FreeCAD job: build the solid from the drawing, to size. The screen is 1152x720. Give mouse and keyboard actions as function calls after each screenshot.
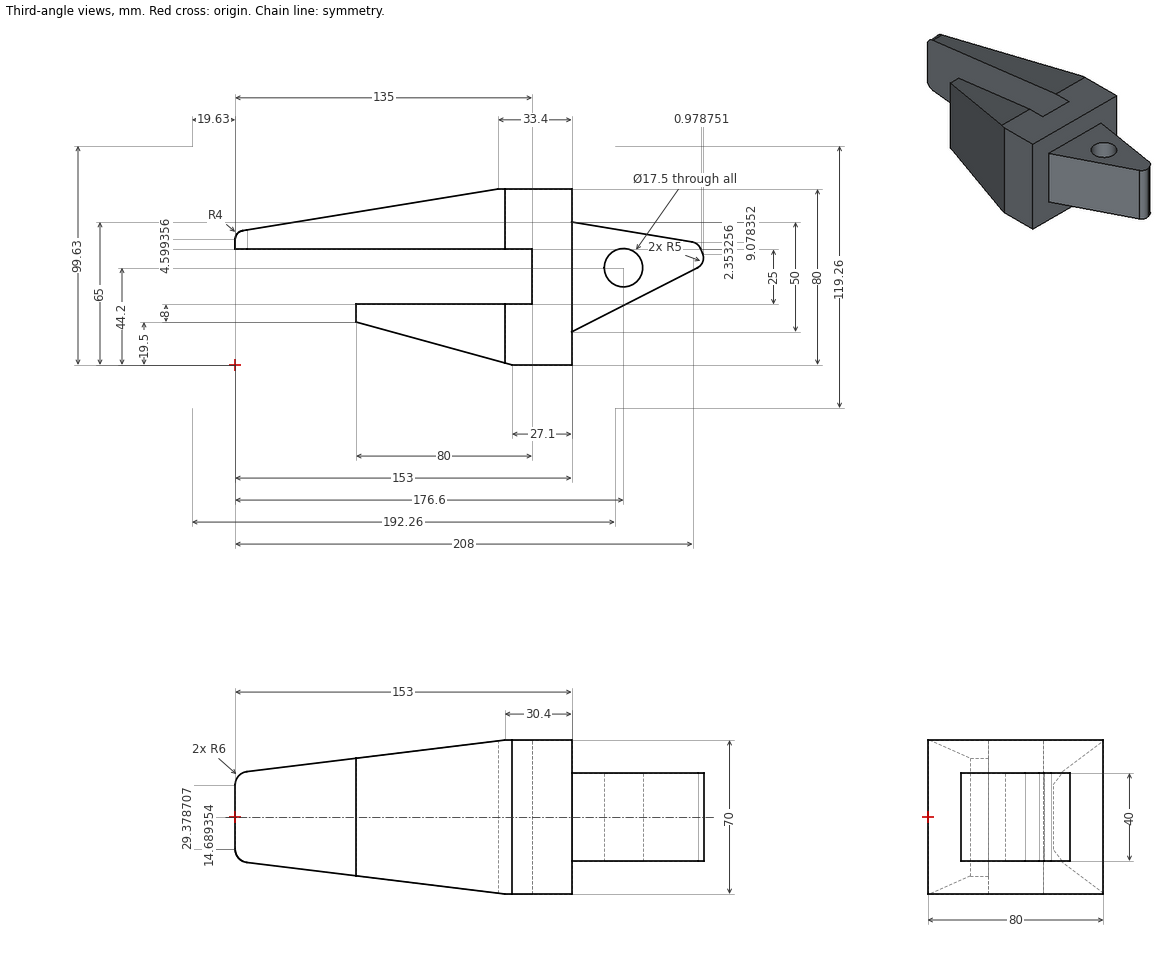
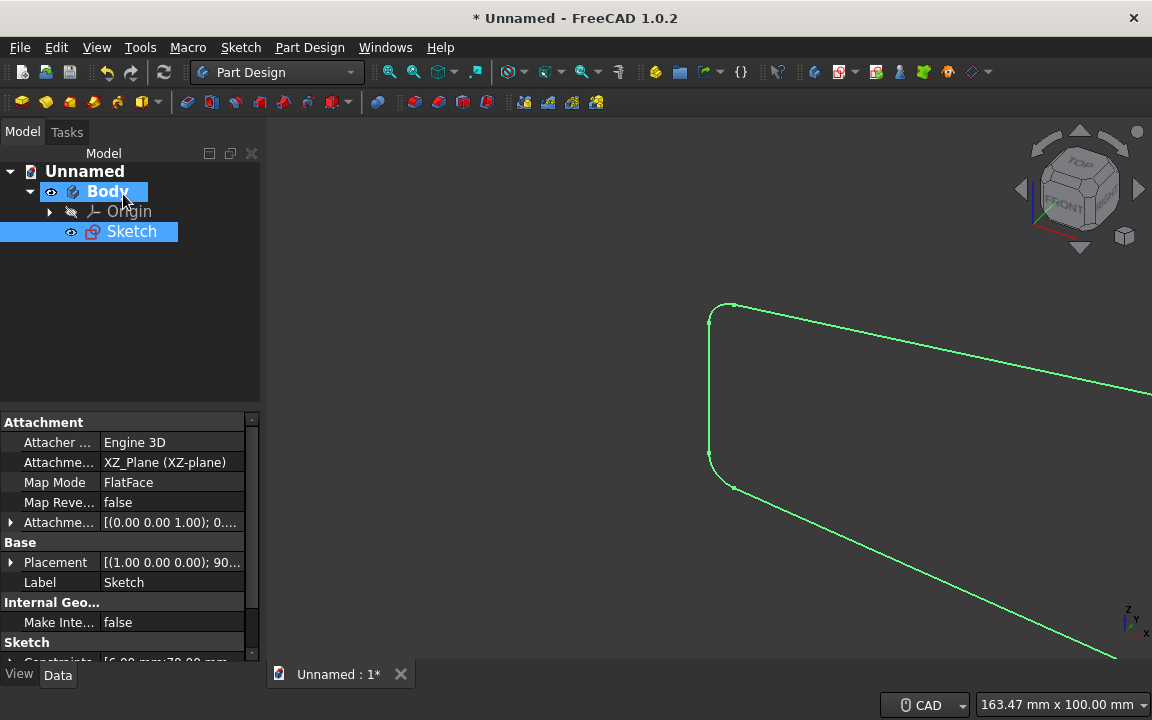
click(22, 102)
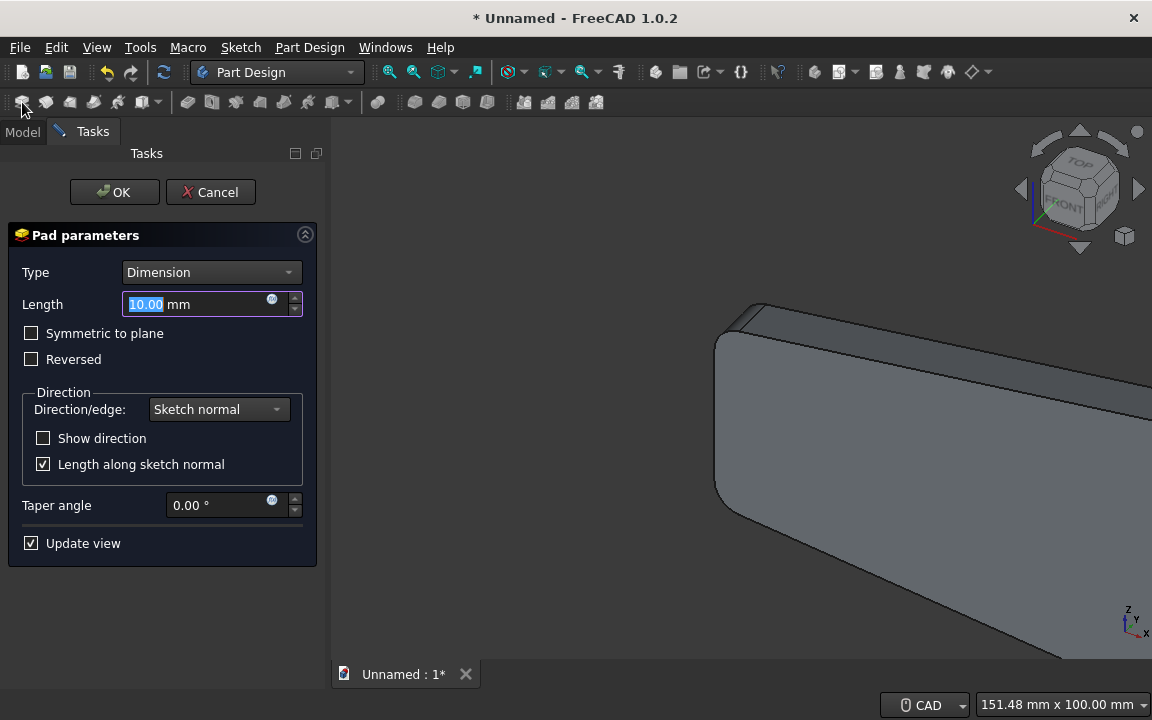
text(80)
key(Tab)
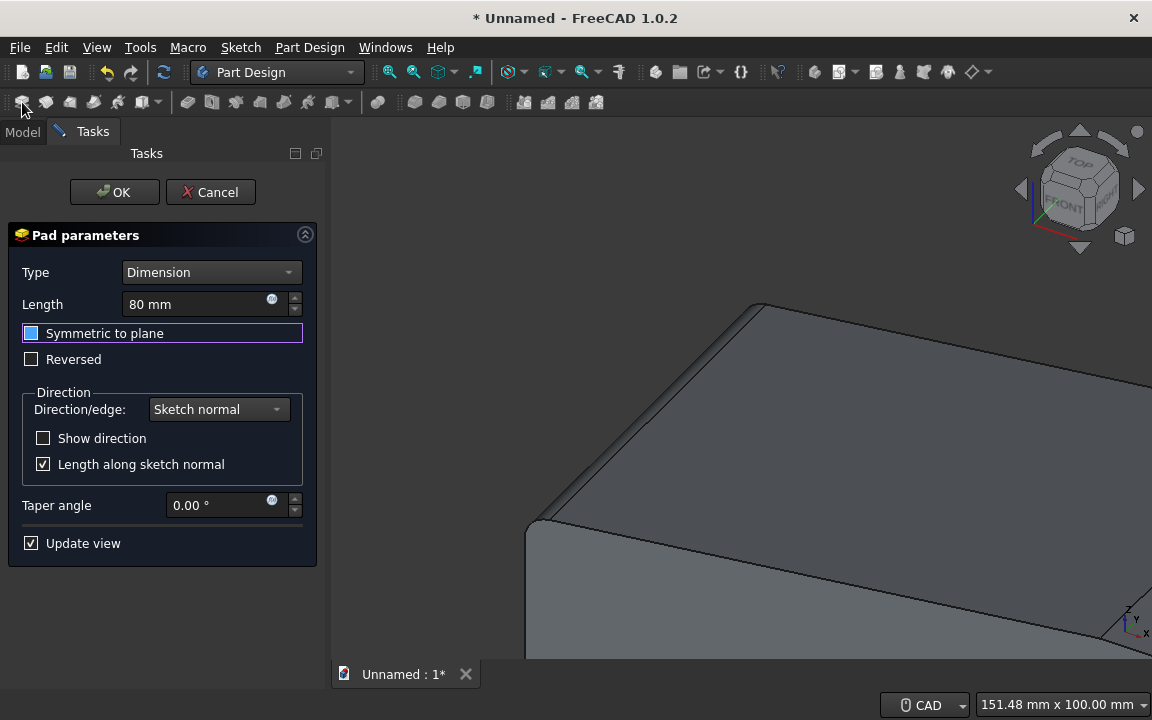
click(30, 359)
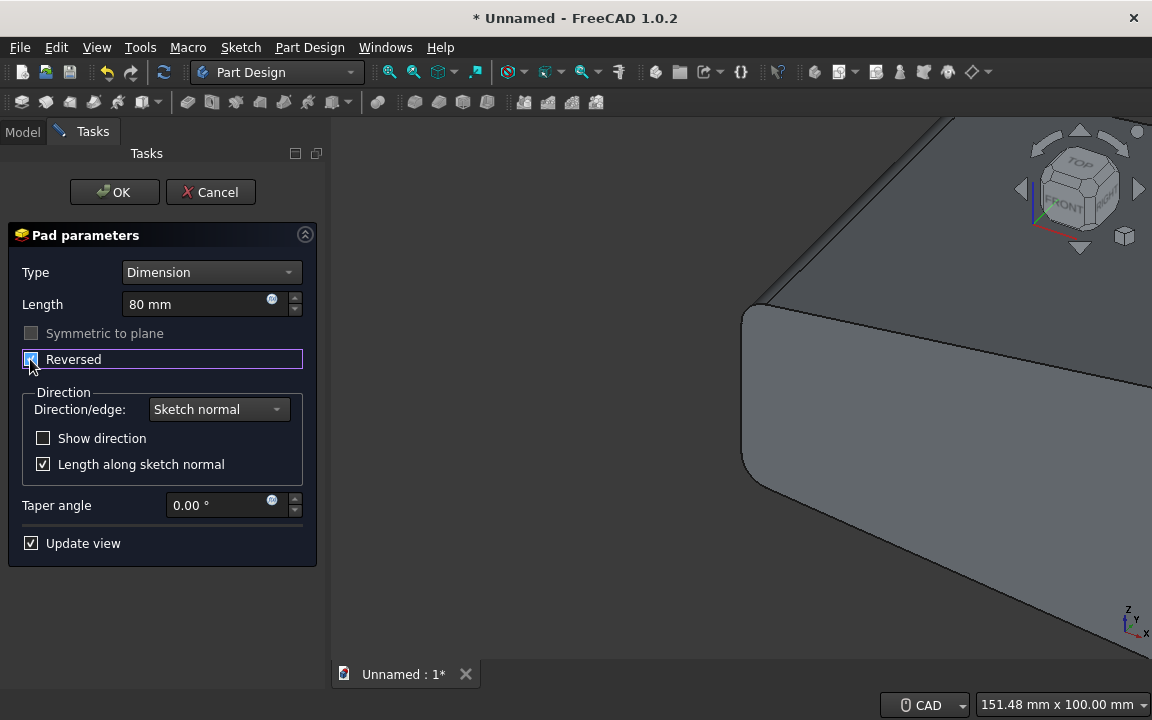
click(115, 192)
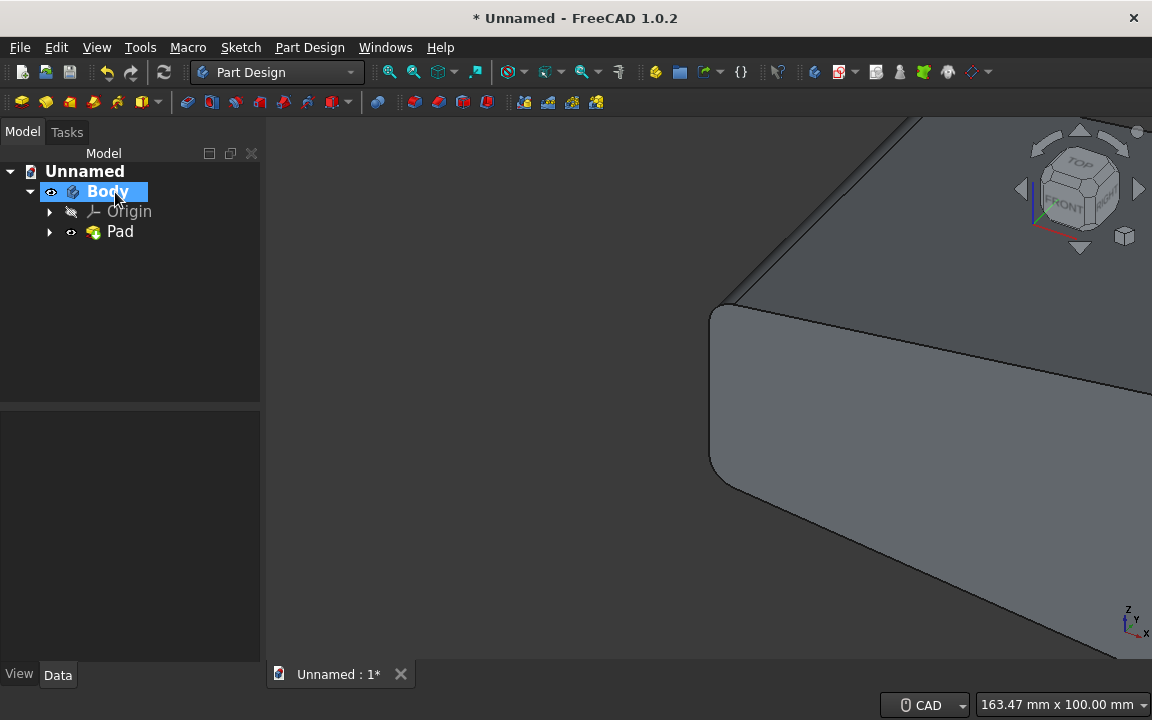
click(390, 72)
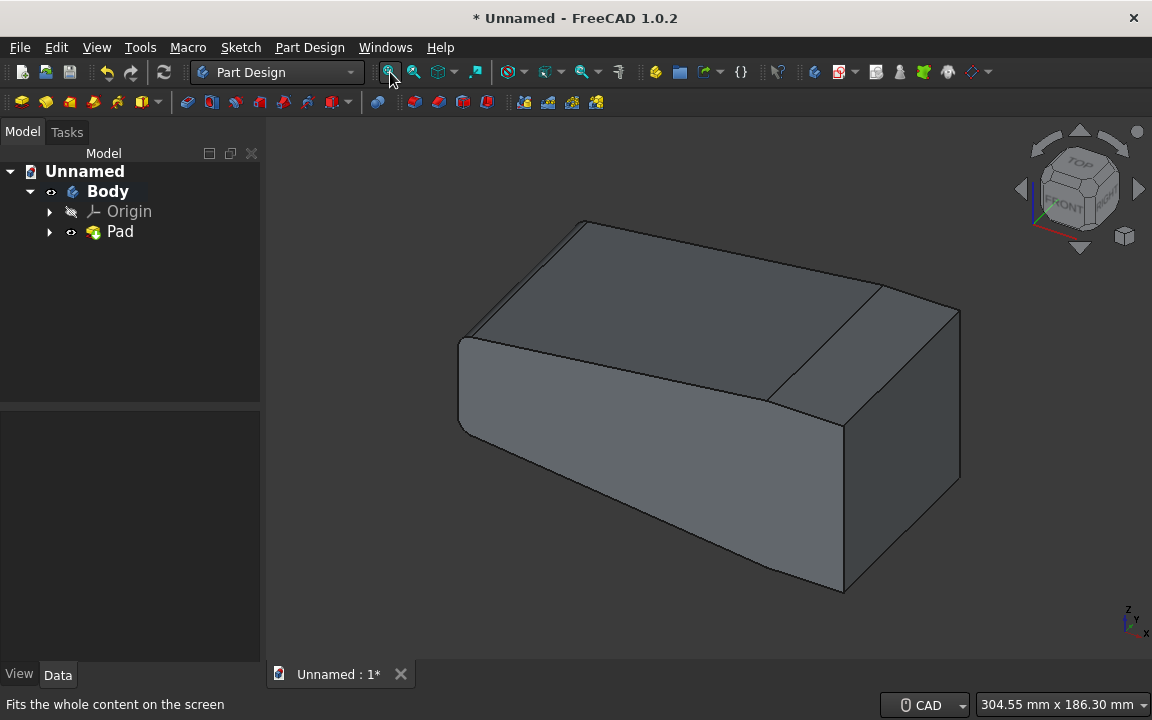
click(840, 72)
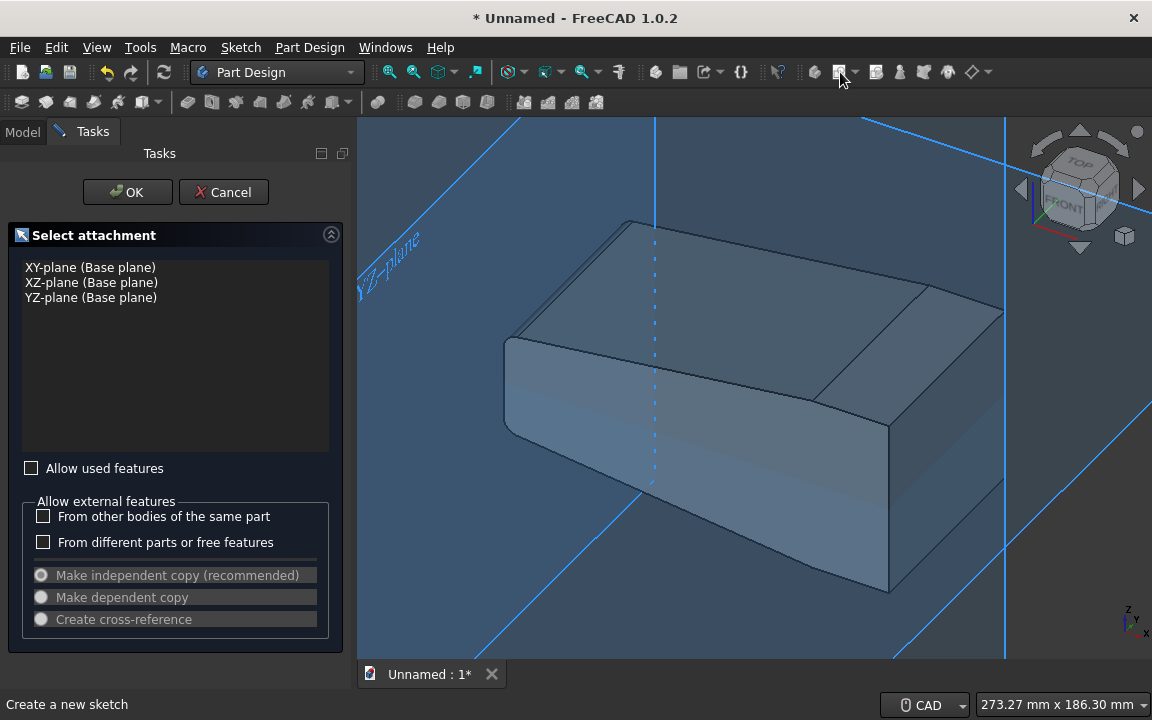
click(82, 268)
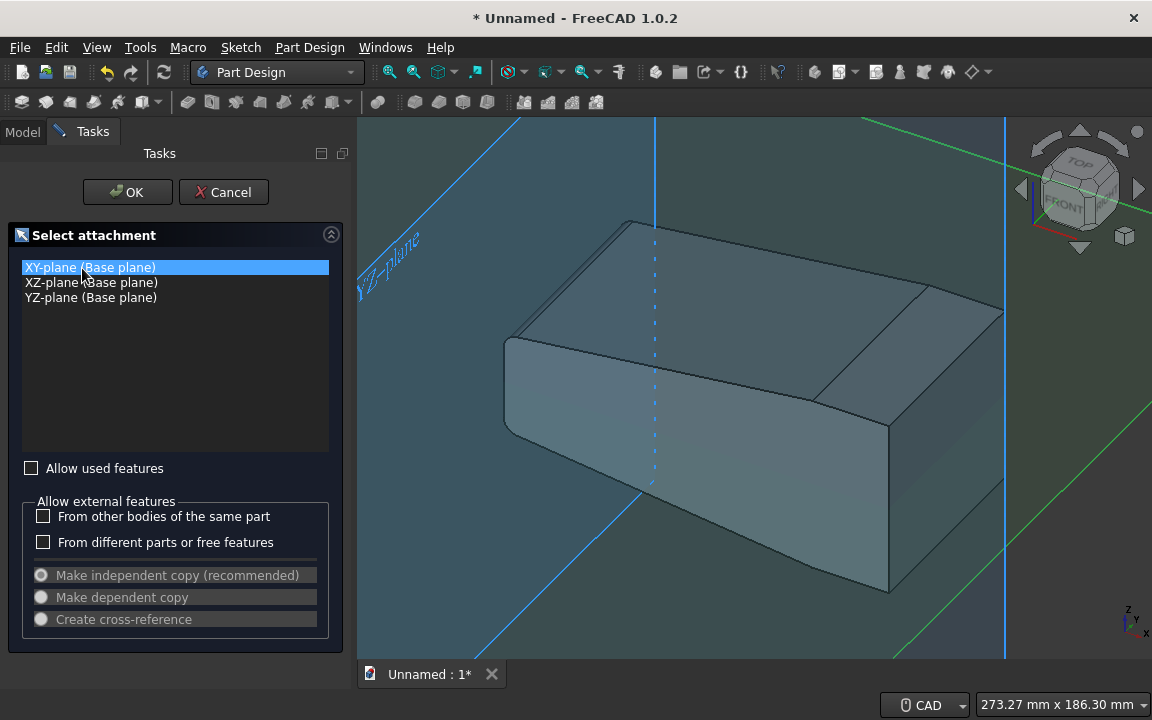
click(128, 192)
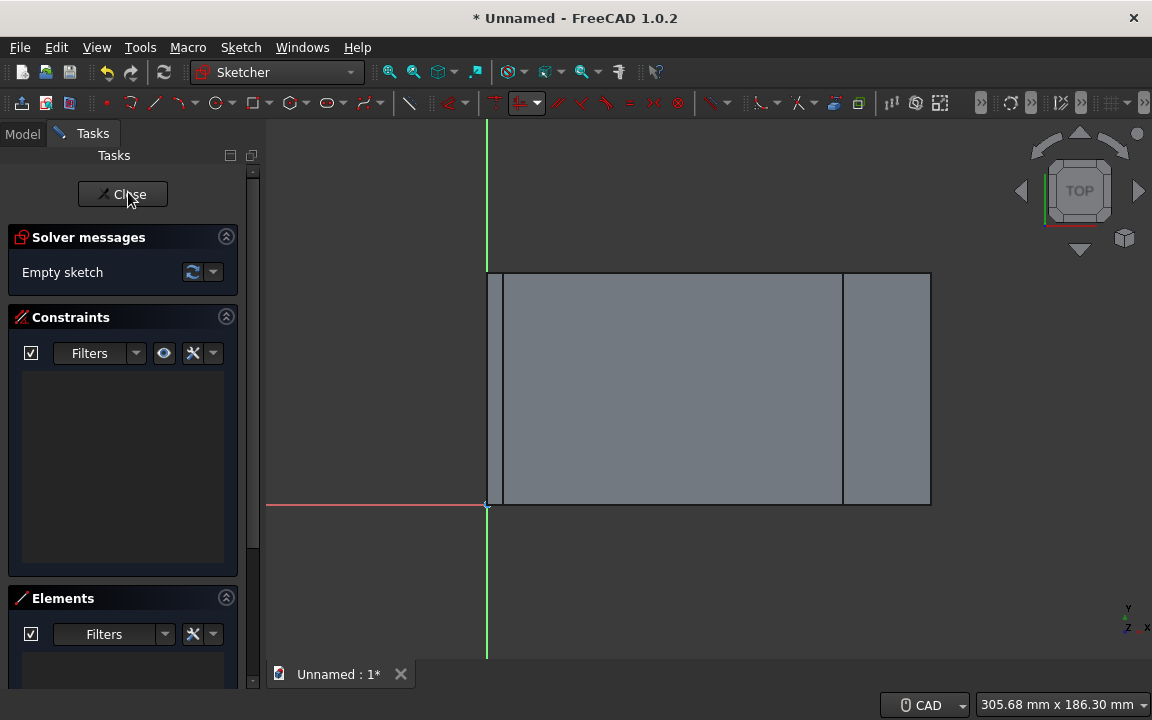
key(q)
key(s)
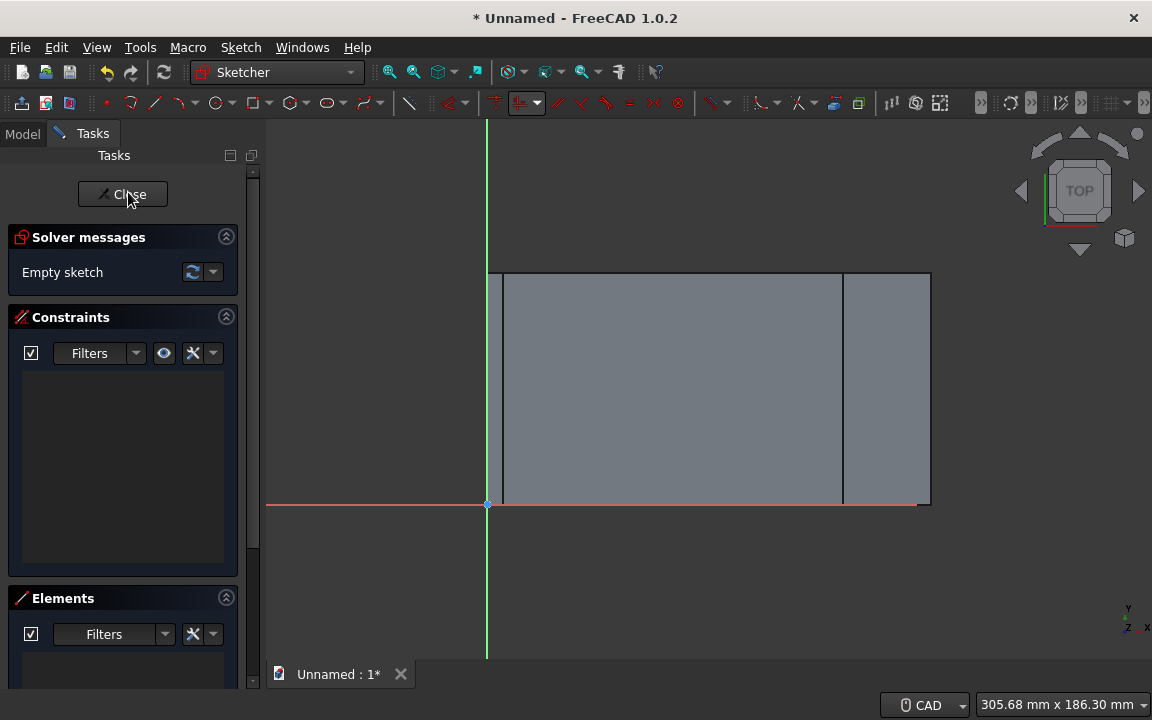
scroll(331, 389, down, 1)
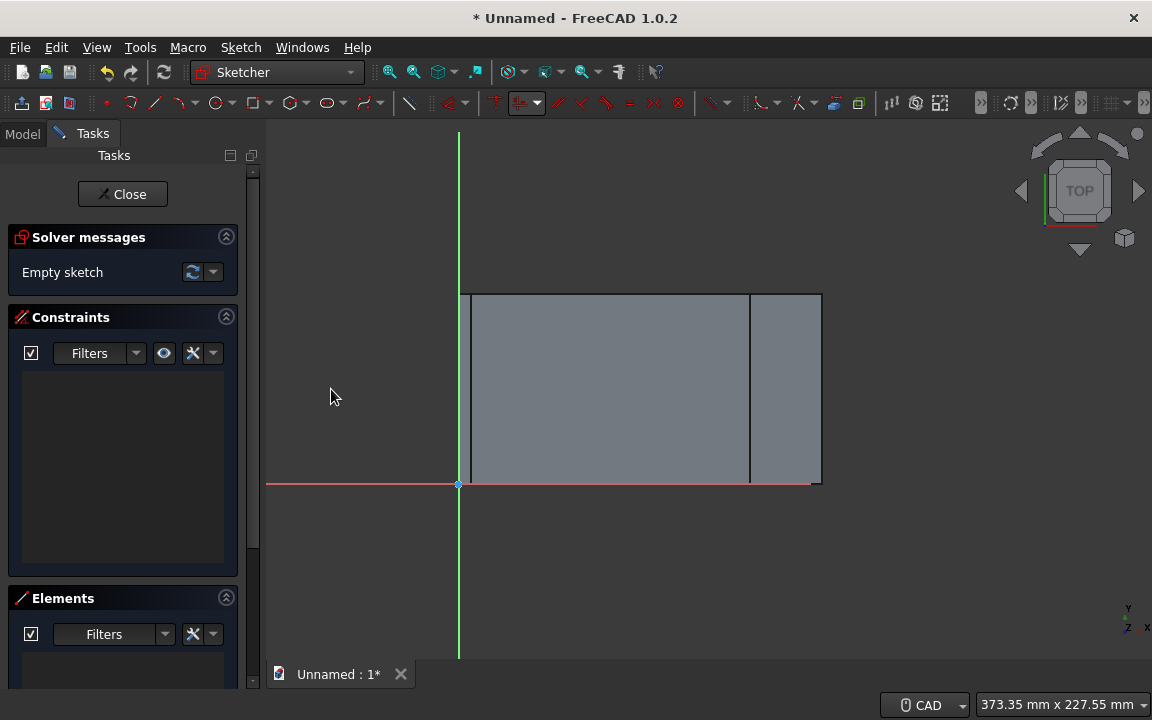
click(254, 104)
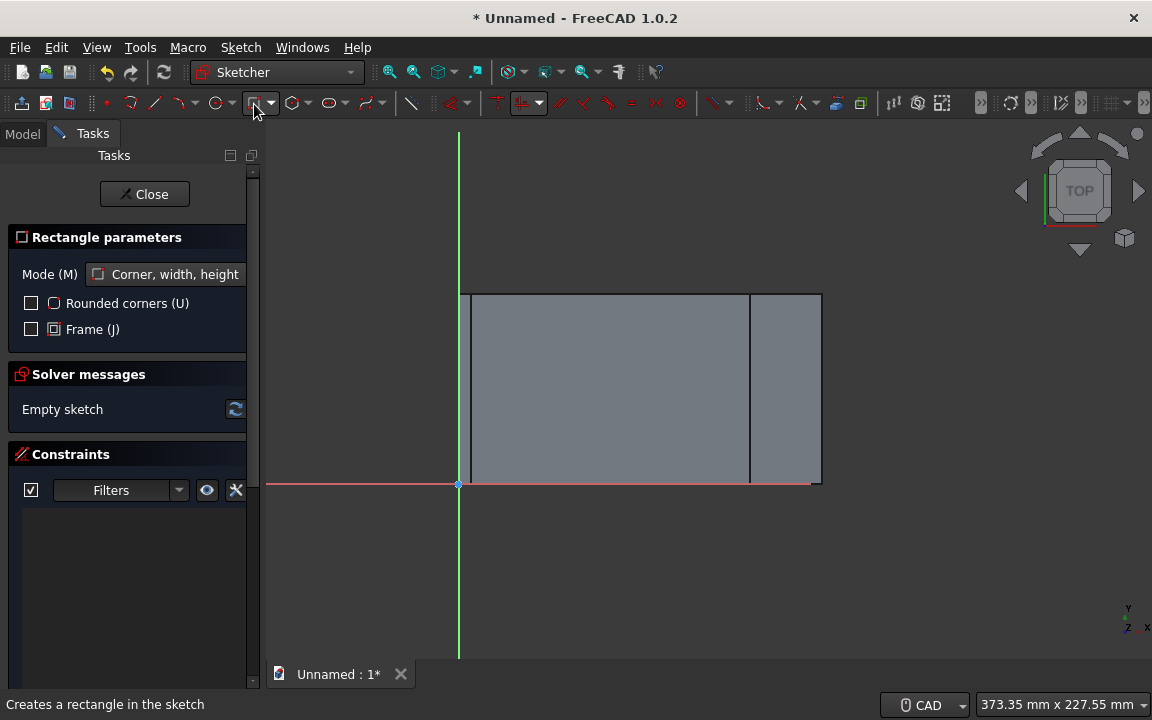
click(412, 248)
move(869, 531)